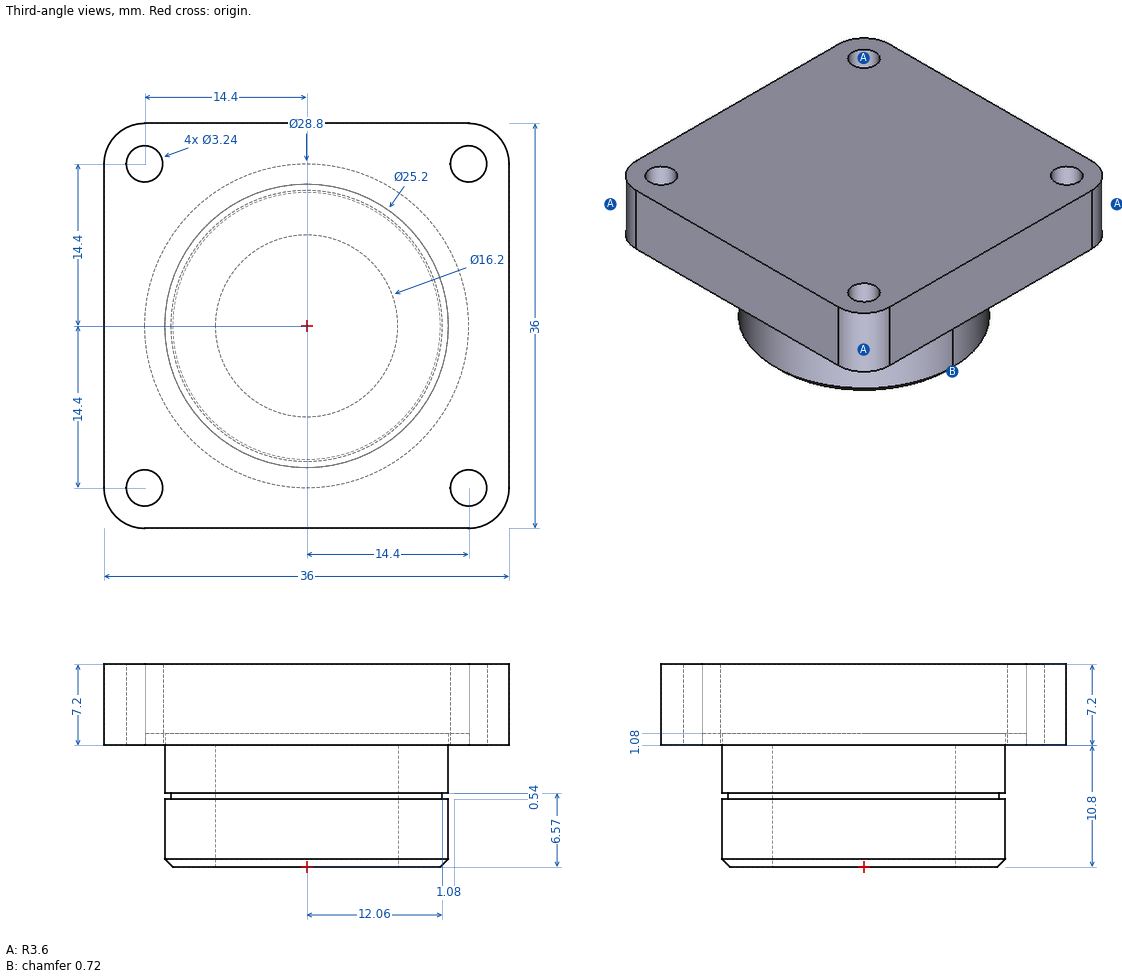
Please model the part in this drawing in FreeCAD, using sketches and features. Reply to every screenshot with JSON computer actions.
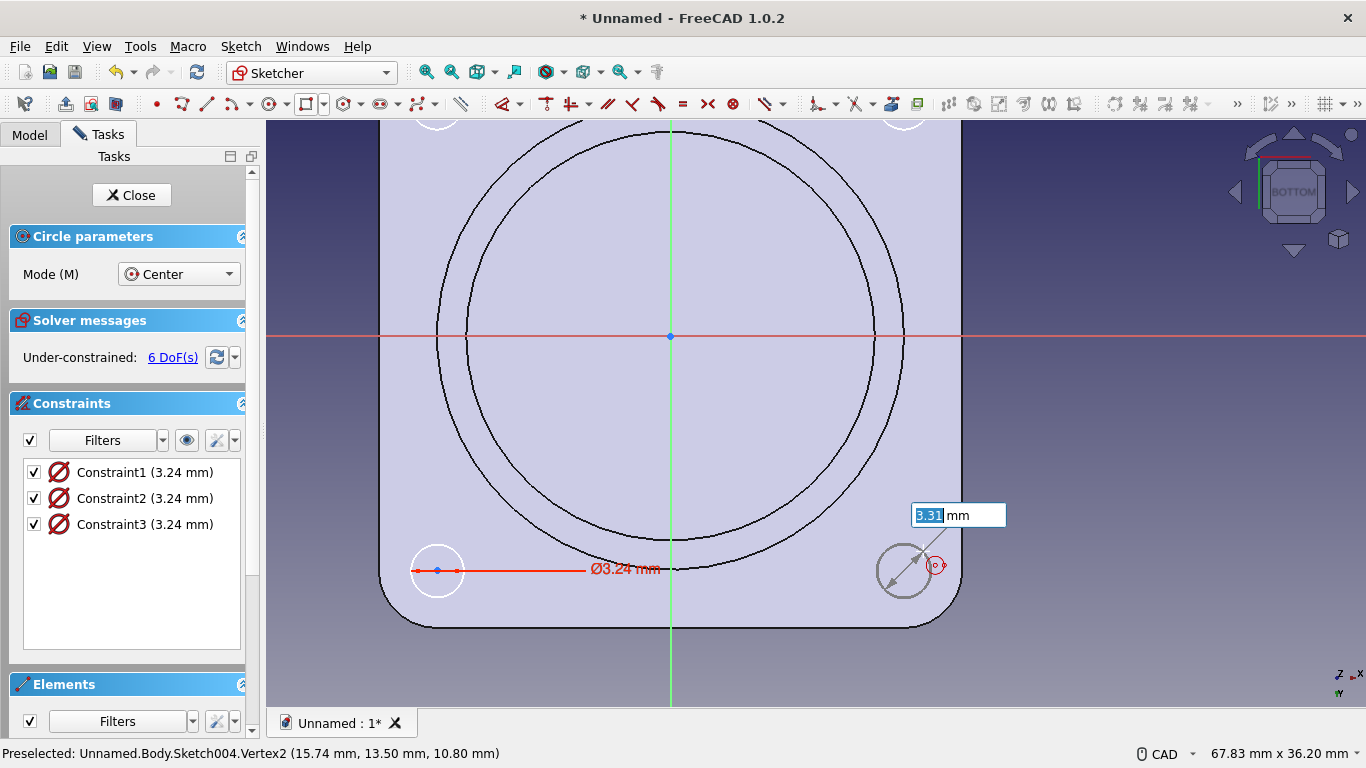
{"action": "type", "text": "3.24"}
{"action": "key", "text": "Return"}
{"action": "key", "text": "Escape"}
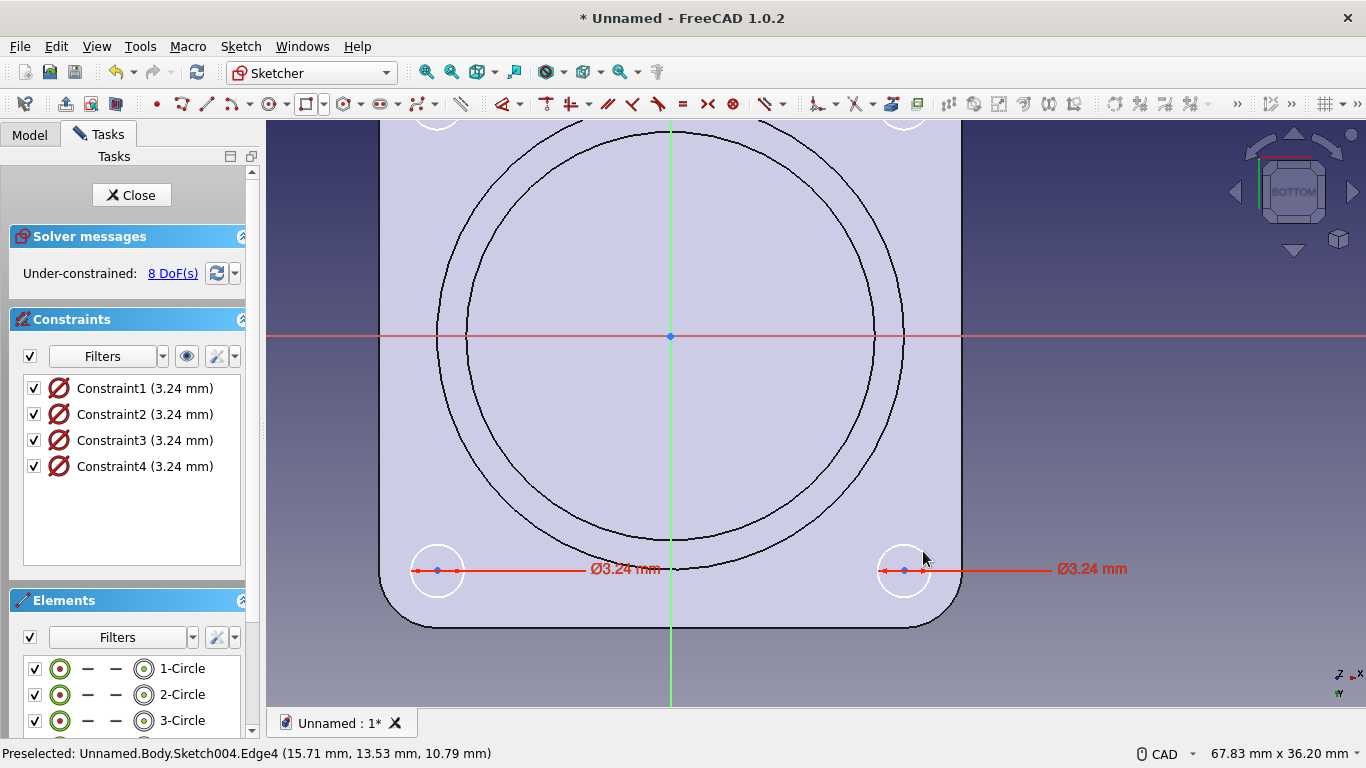
{"action": "left_click", "coordinate": [437, 571]}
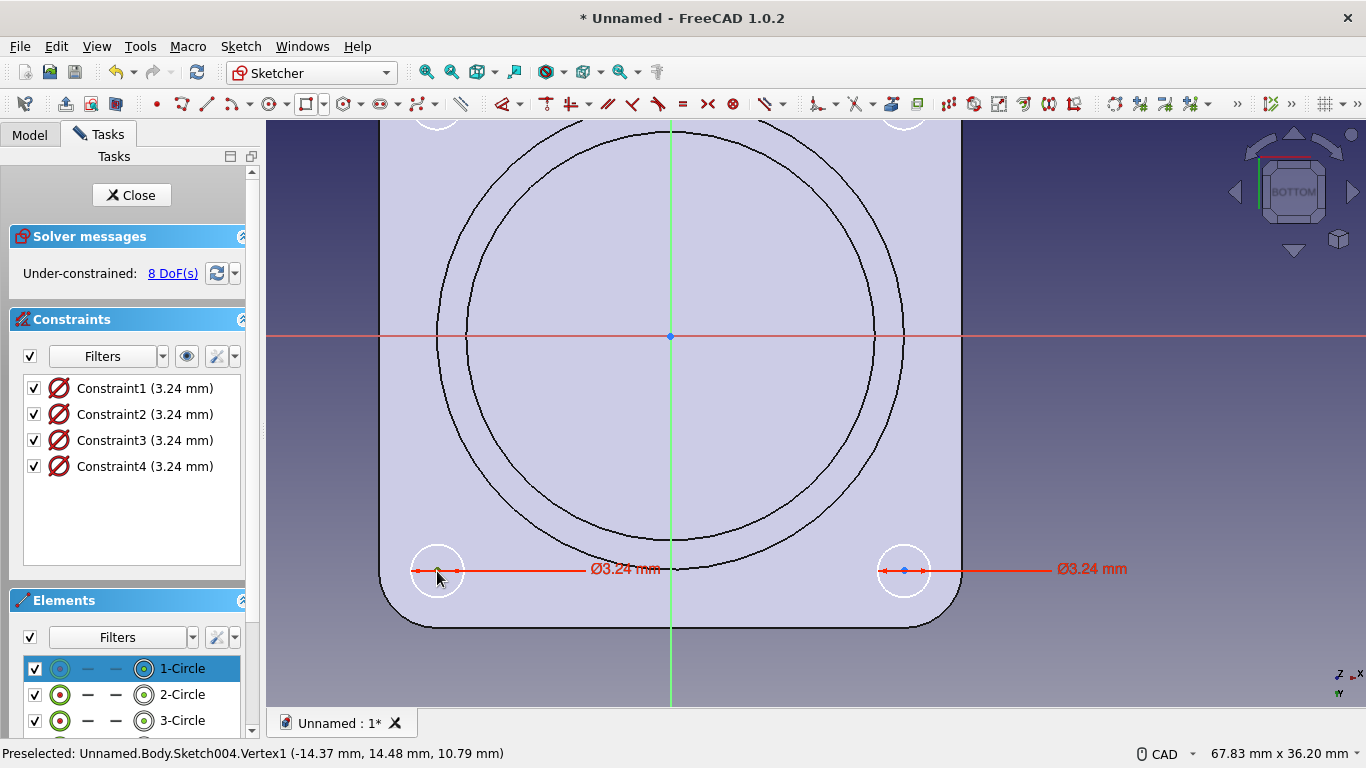
{"action": "scroll", "coordinate": [904, 571], "scroll_direction": "down", "scroll_amount": 2}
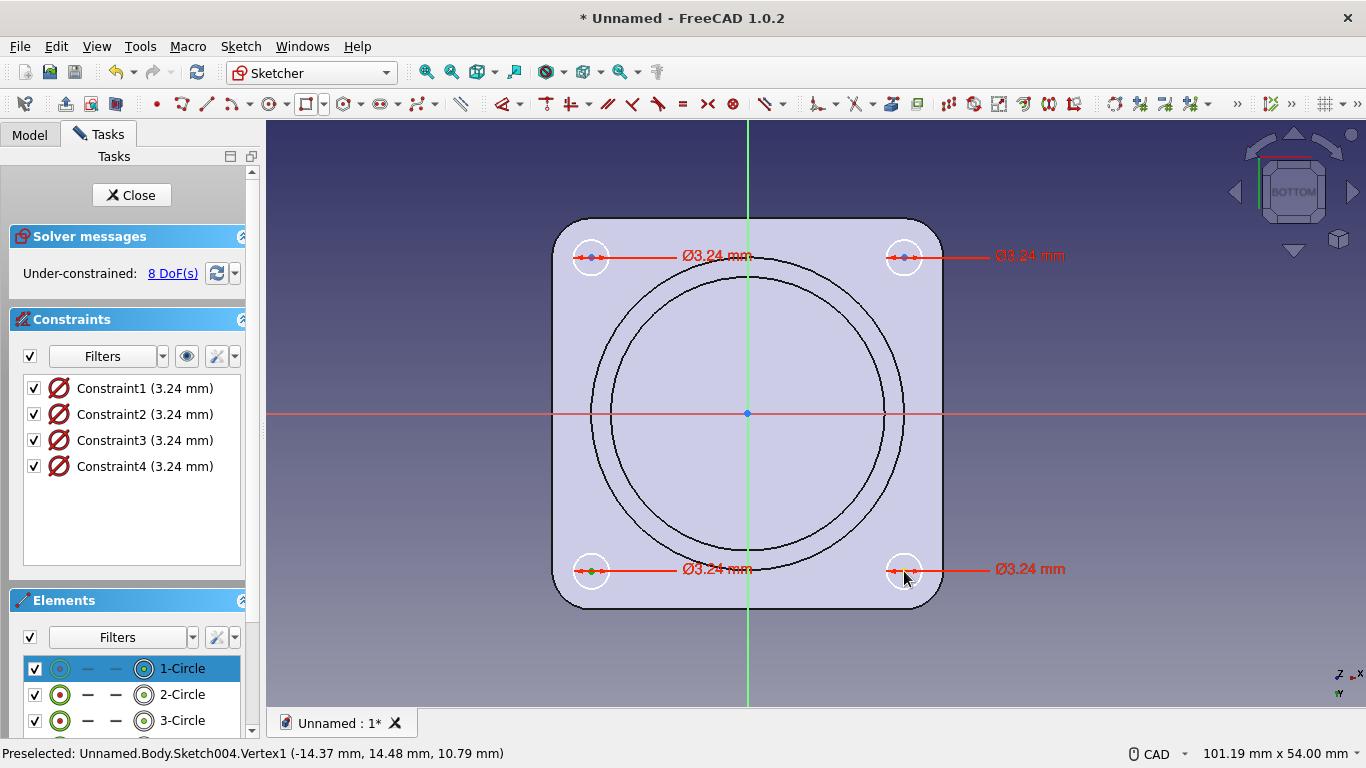
{"action": "left_click", "coordinate": [591, 258]}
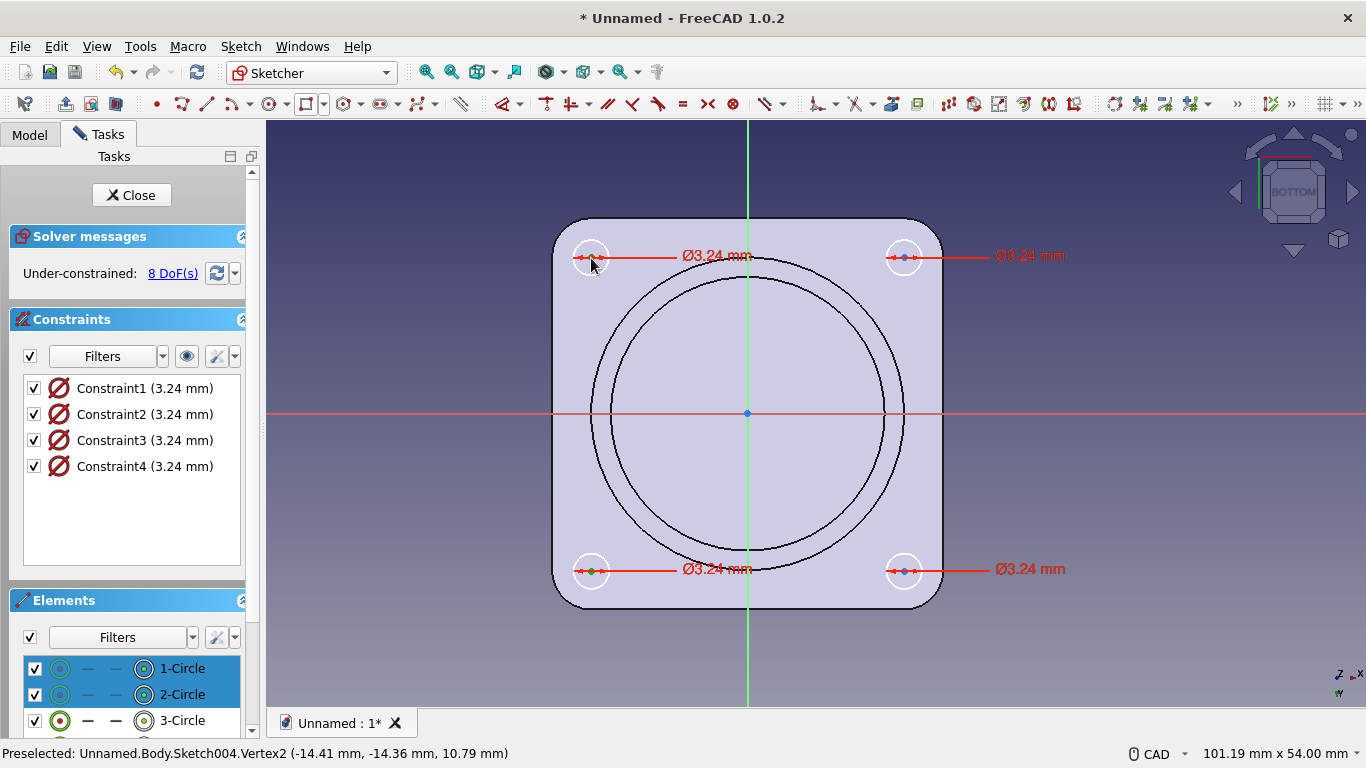
{"action": "key", "text": "v"}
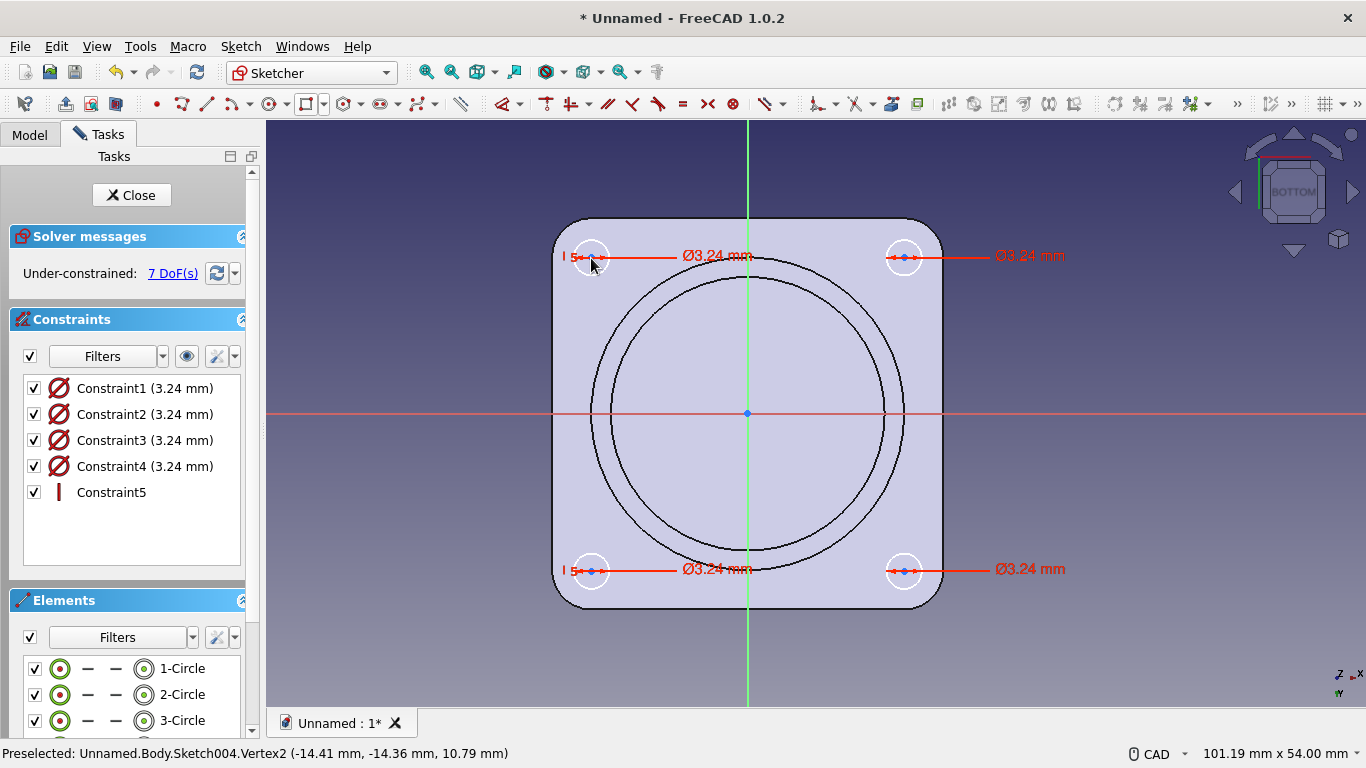
{"action": "left_click", "coordinate": [591, 258]}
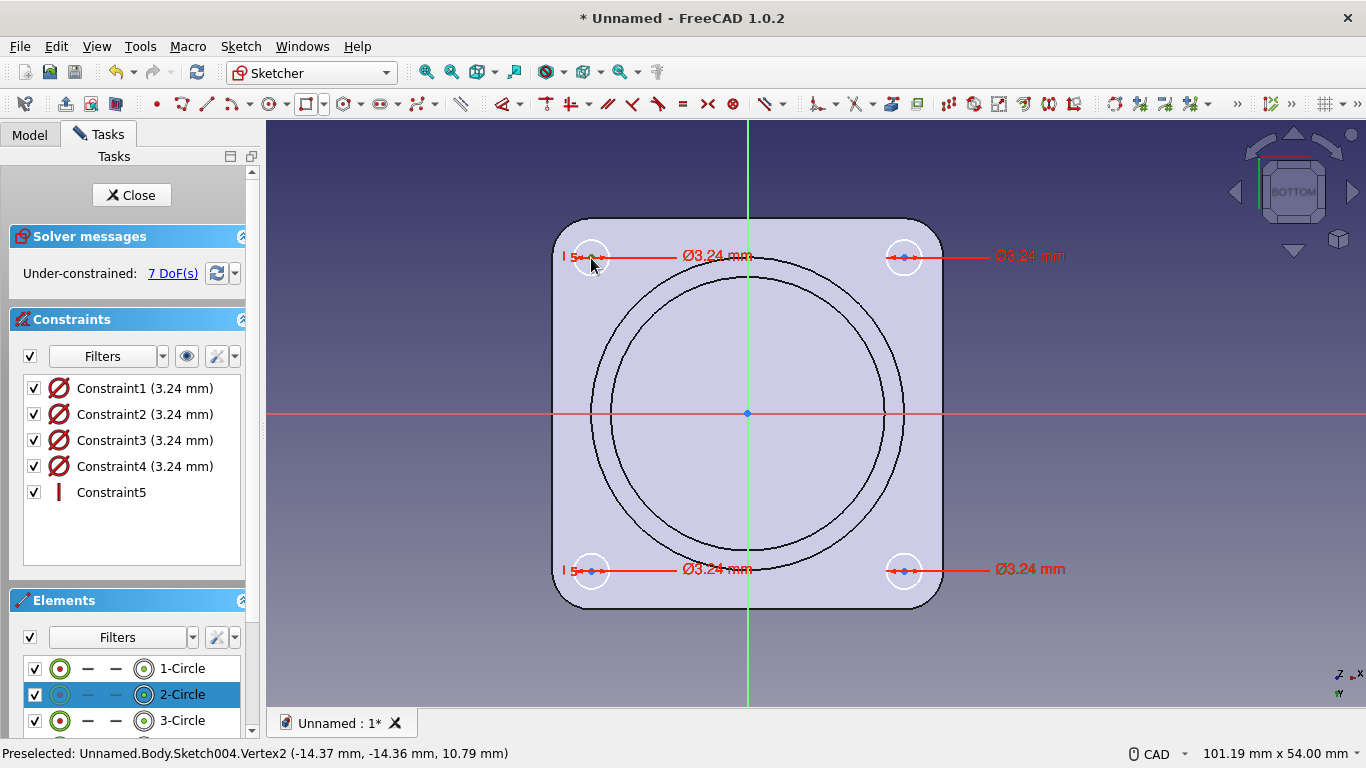
{"action": "left_click", "coordinate": [904, 258]}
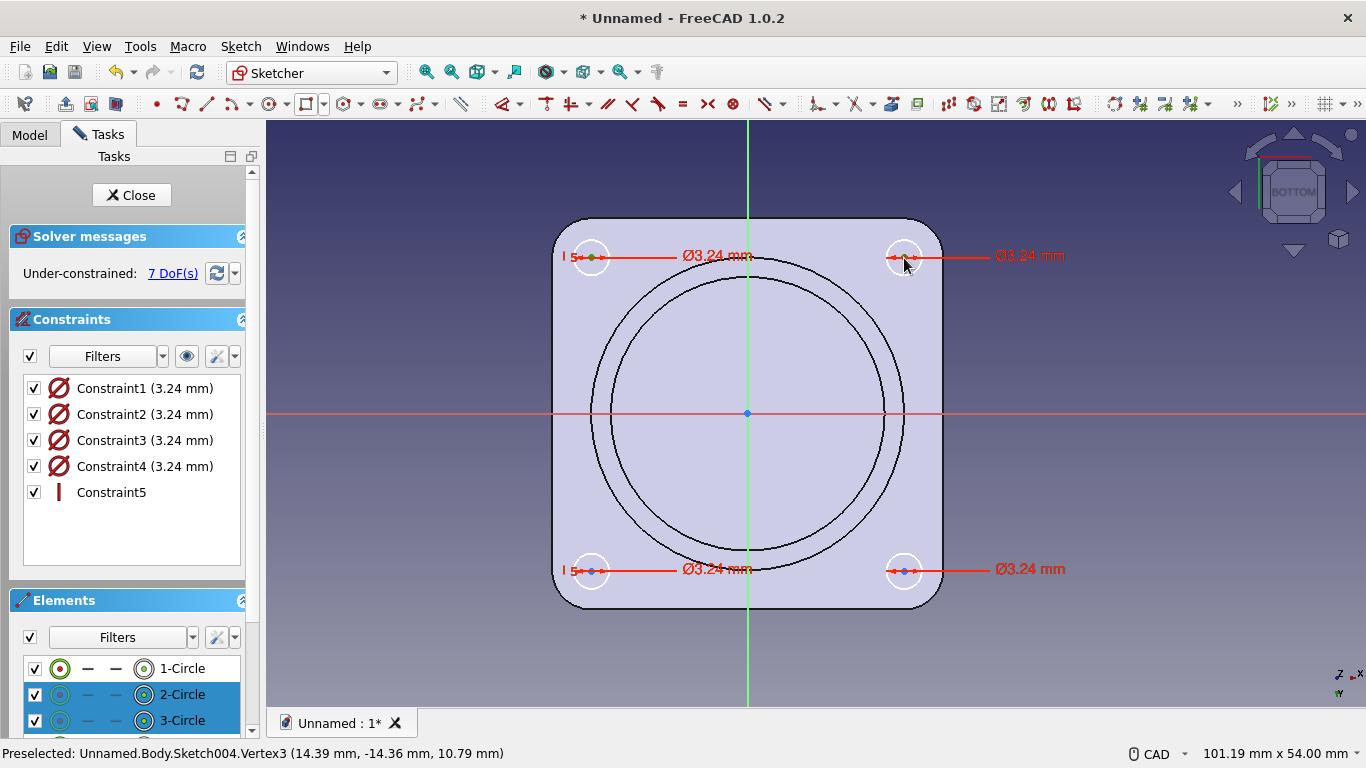
{"action": "key", "text": "h"}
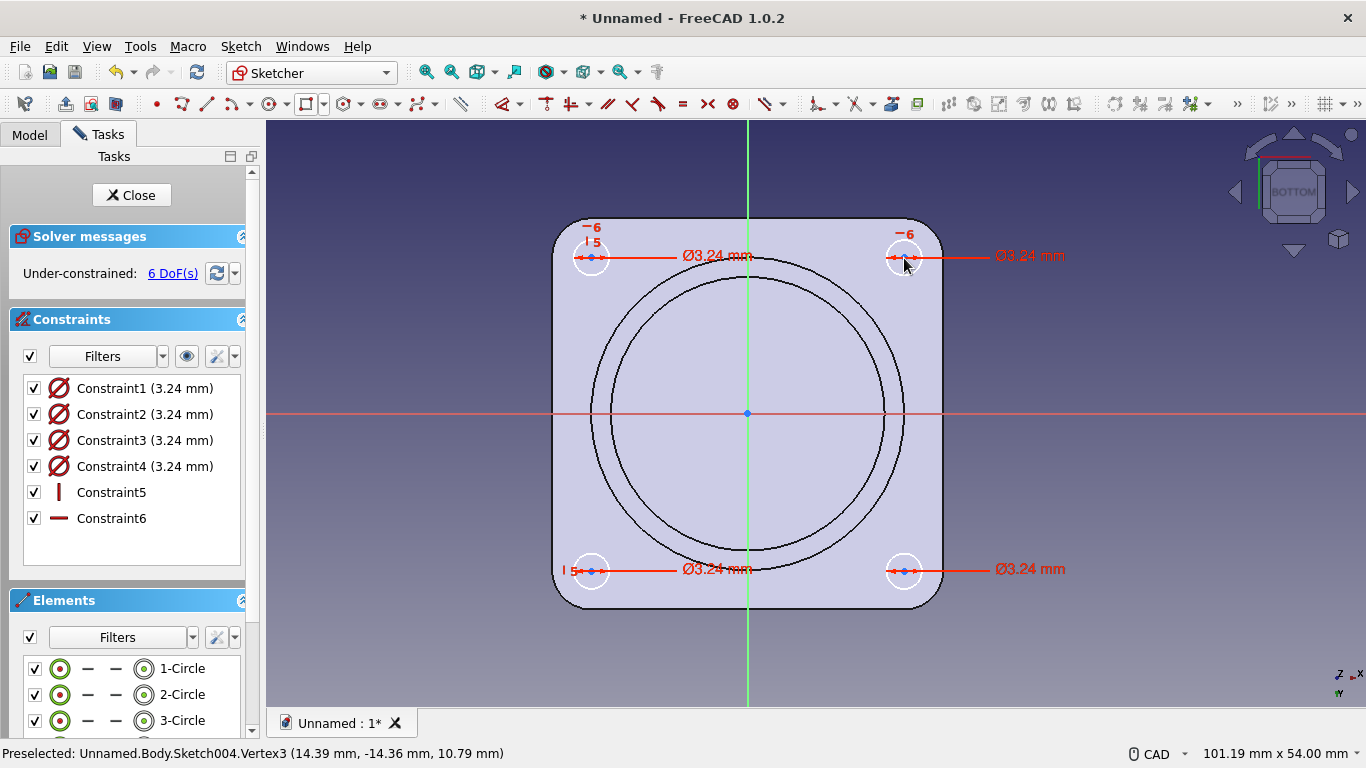
{"action": "left_click", "coordinate": [904, 258]}